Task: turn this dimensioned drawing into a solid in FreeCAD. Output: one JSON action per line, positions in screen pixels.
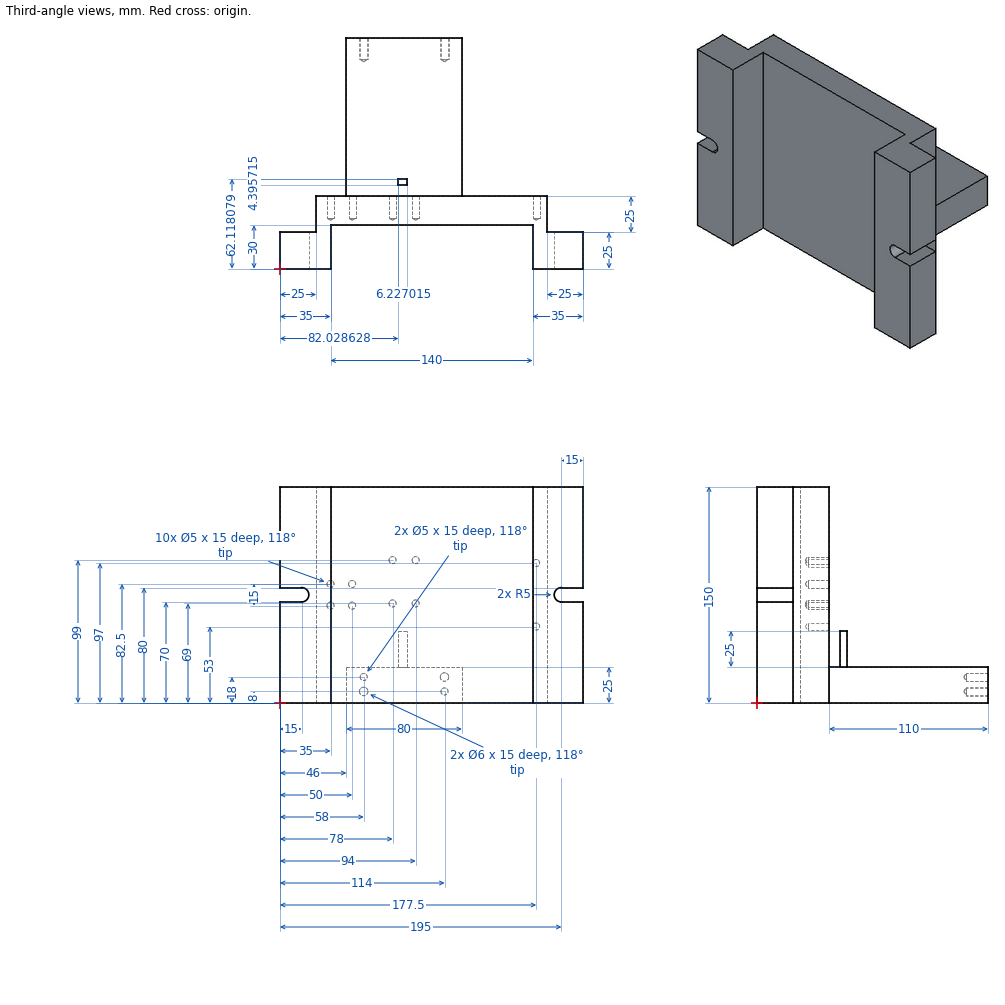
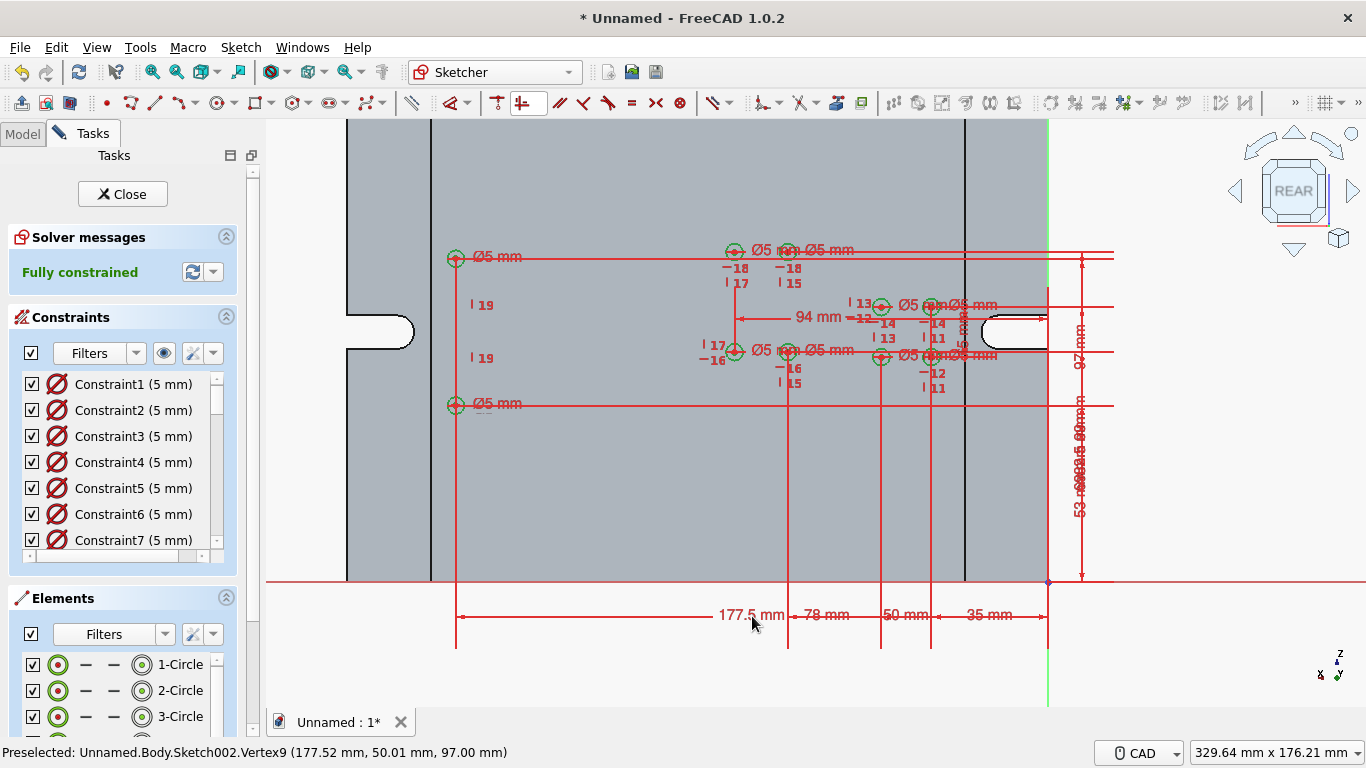
{"action": "left_click", "coordinate": [123, 194]}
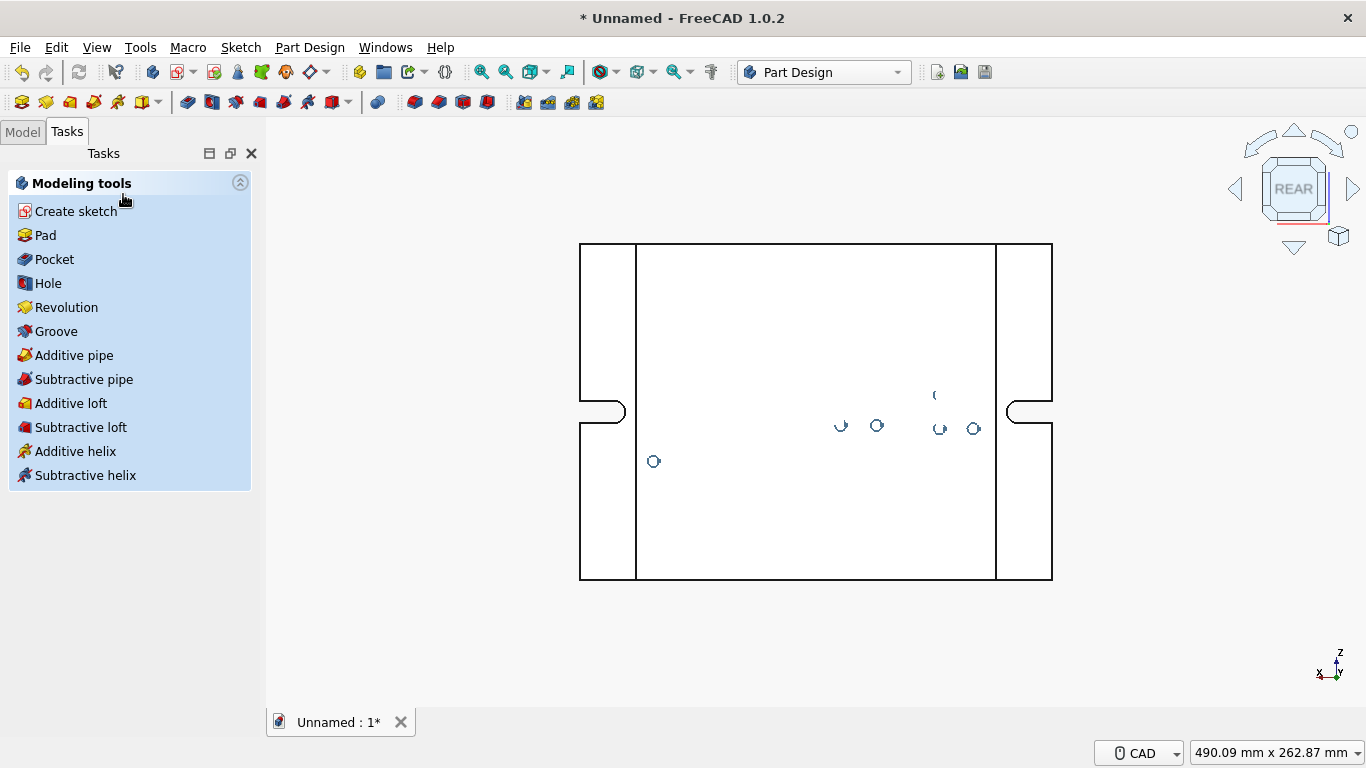
{"action": "left_click", "coordinate": [212, 102]}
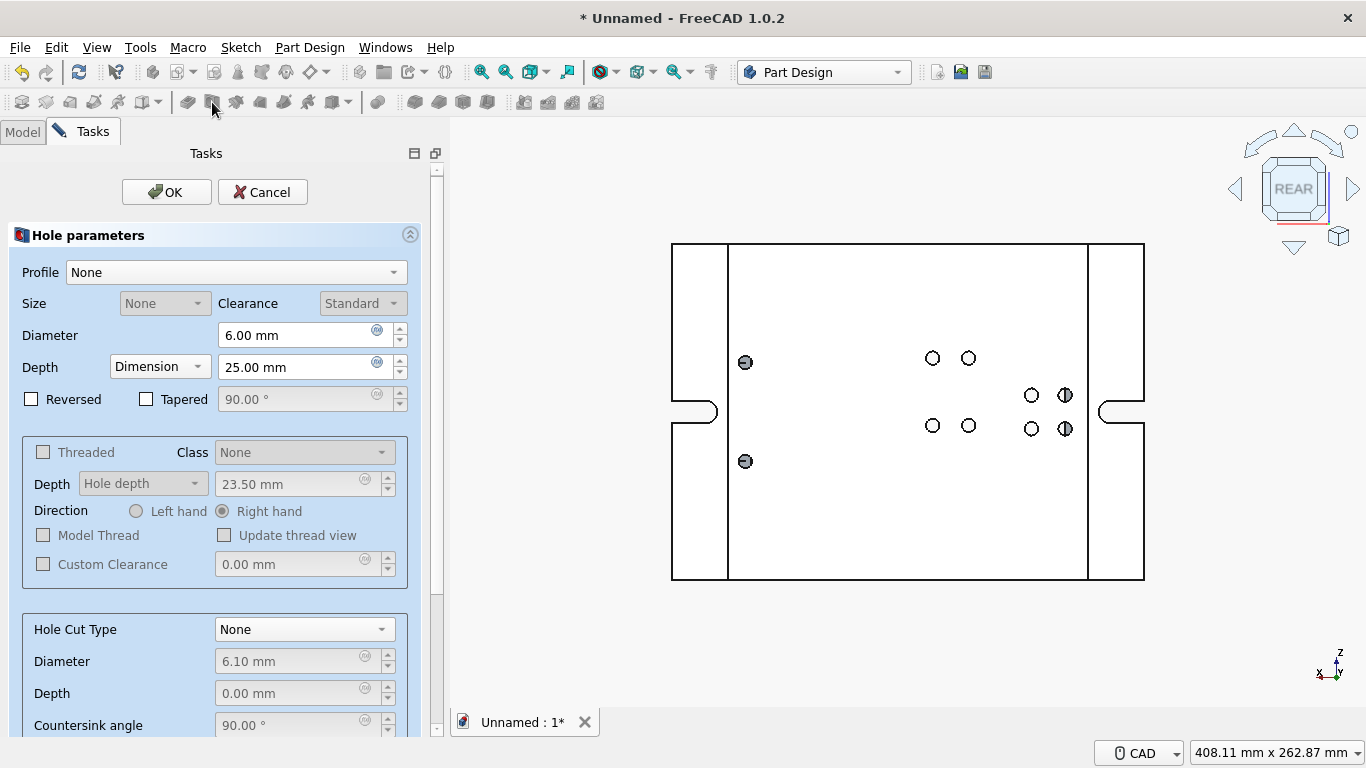
{"action": "triple_click", "coordinate": [305, 335]}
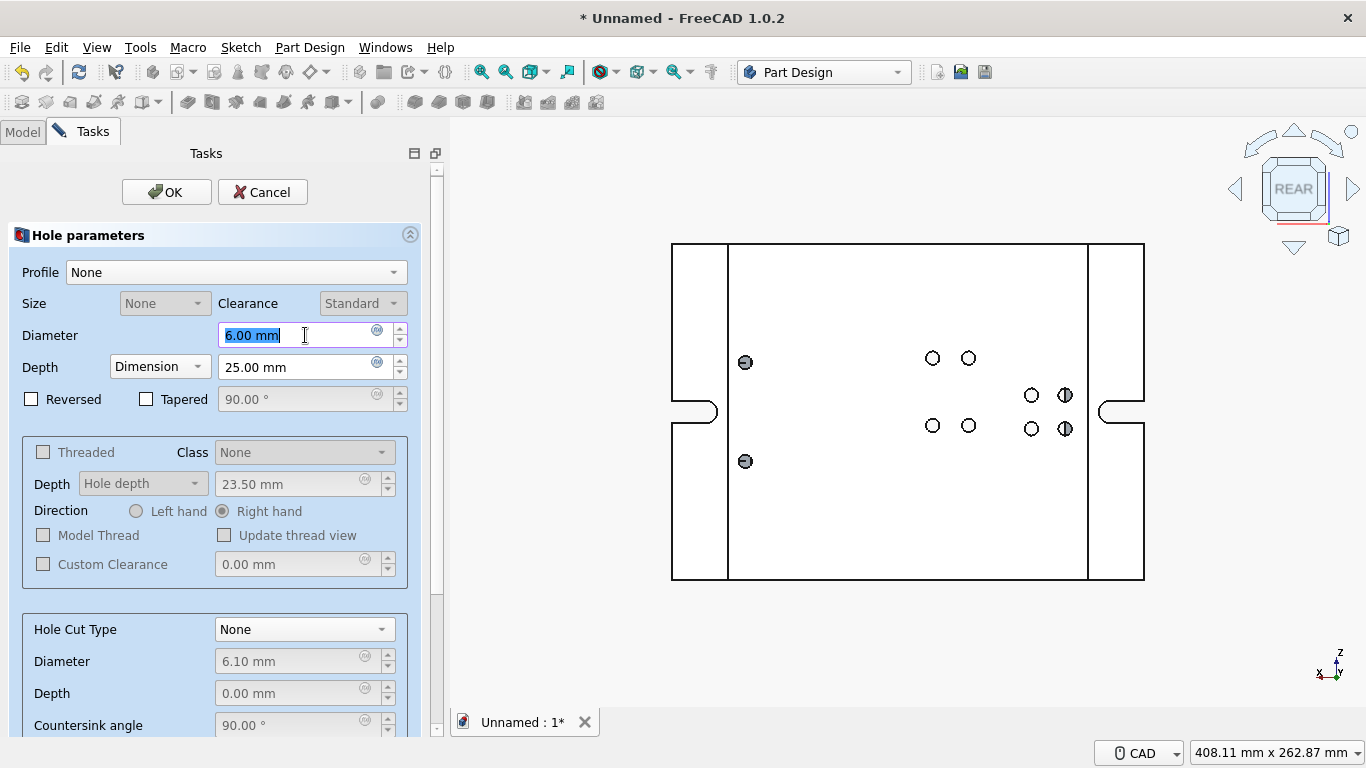
{"action": "type", "text": "5"}
{"action": "key", "text": "Tab"}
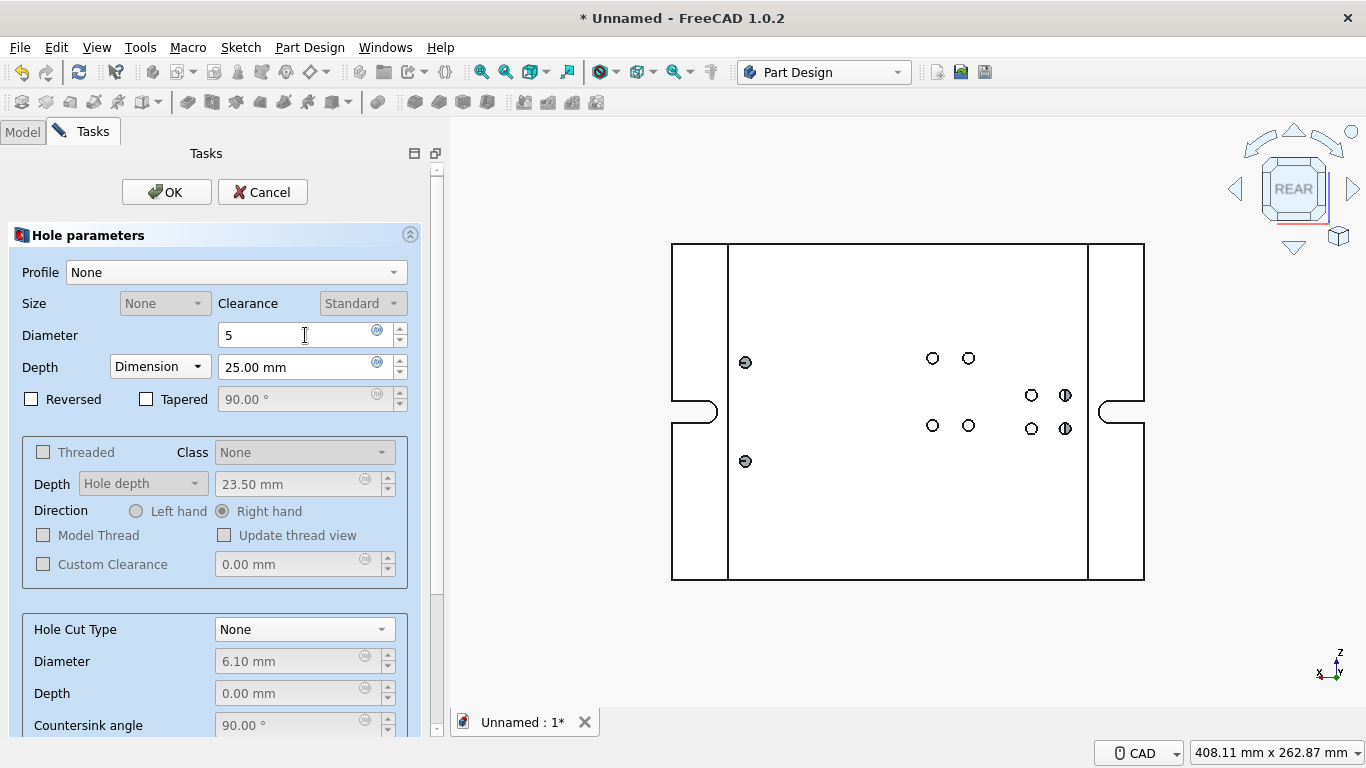
{"action": "triple_click", "coordinate": [305, 367]}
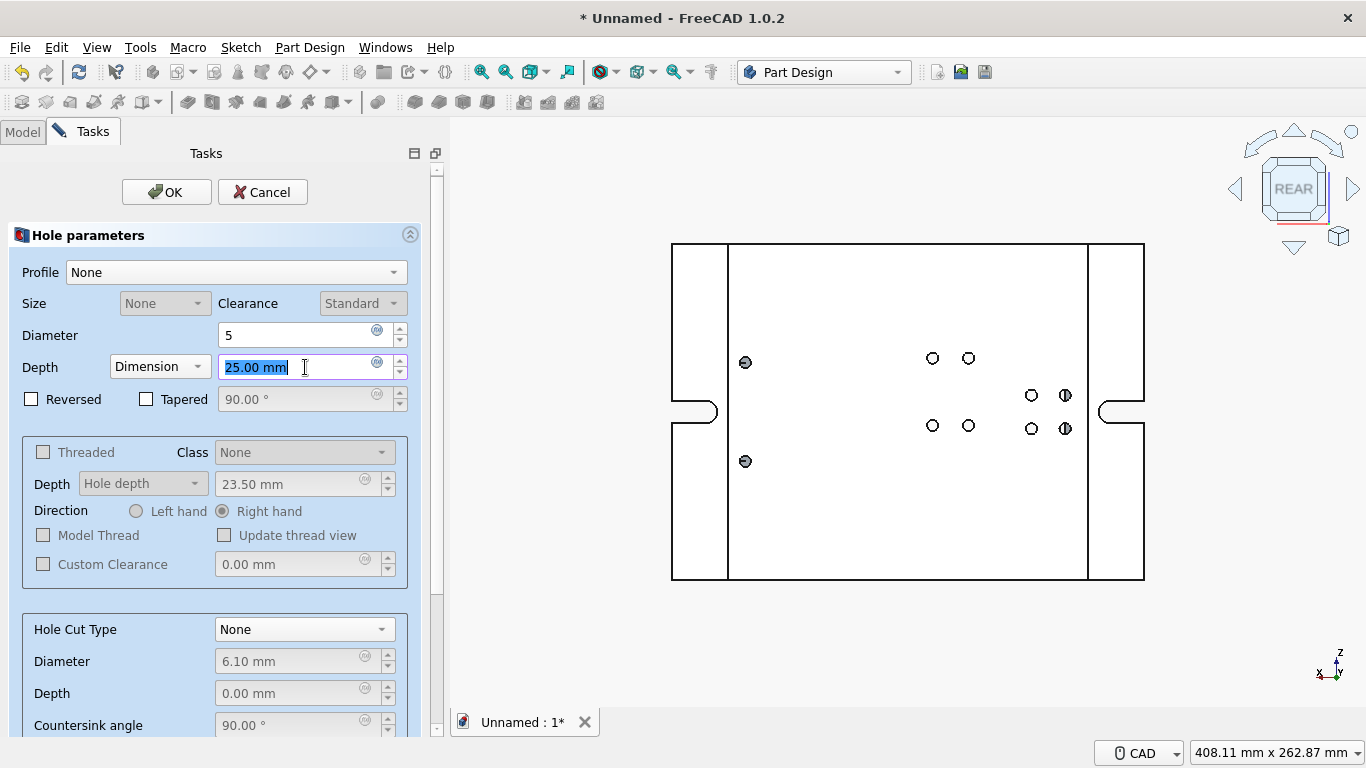
{"action": "type", "text": "15"}
{"action": "key", "text": "Tab"}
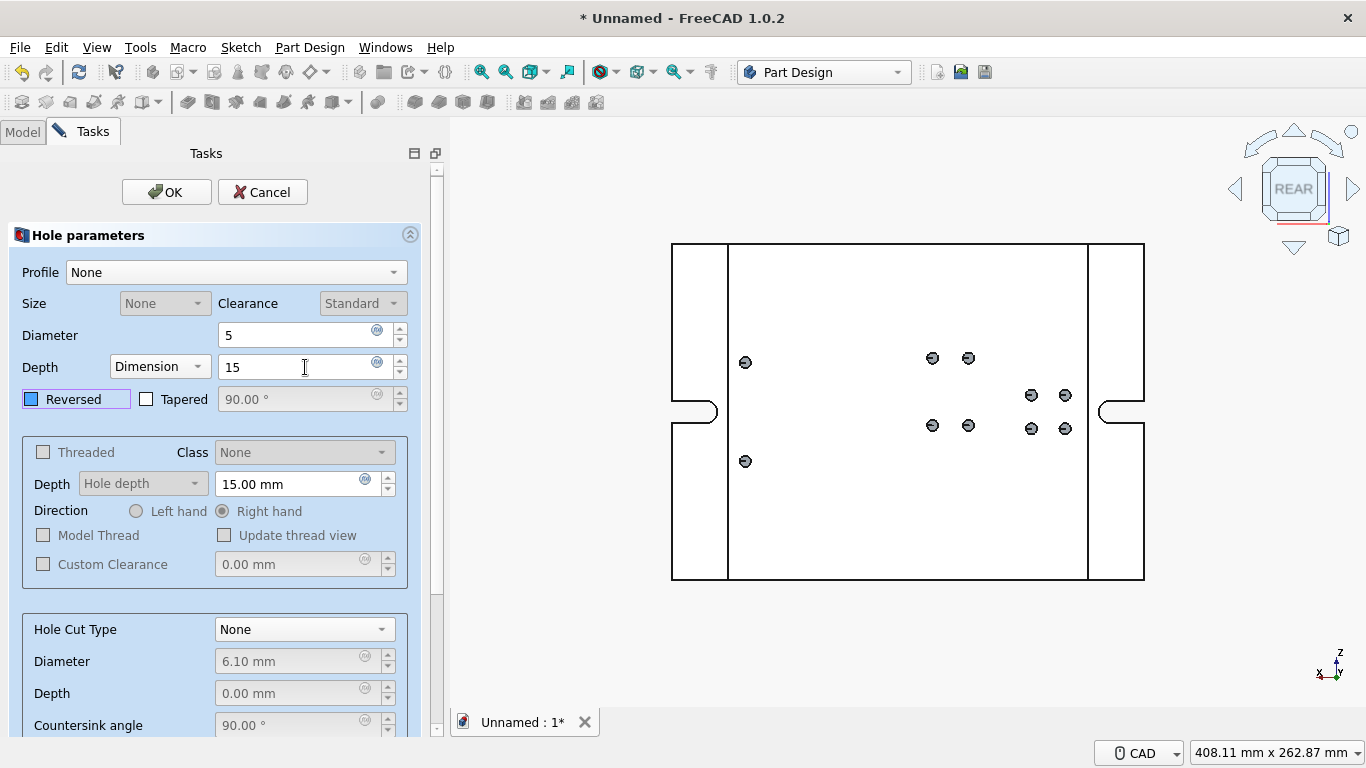
{"action": "left_click", "coordinate": [167, 192]}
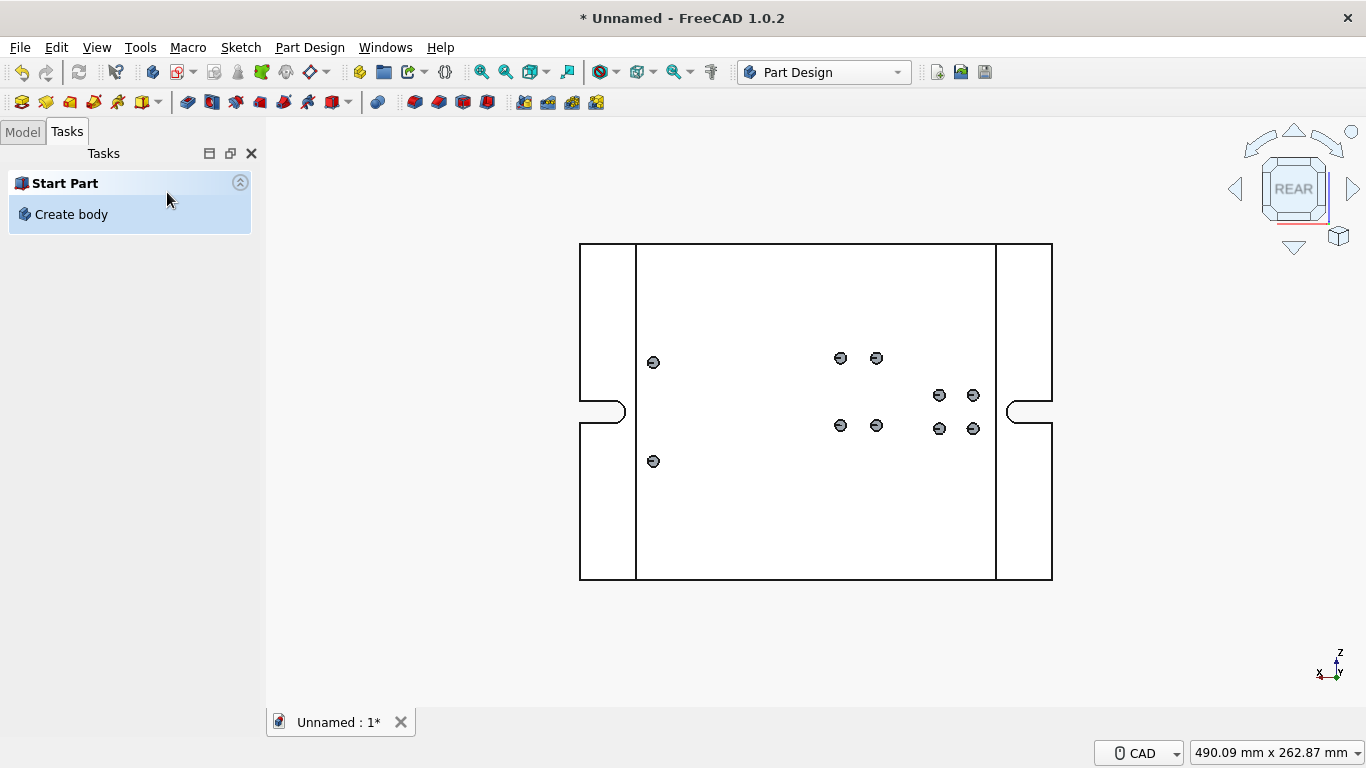
{"action": "left_click", "coordinate": [765, 459]}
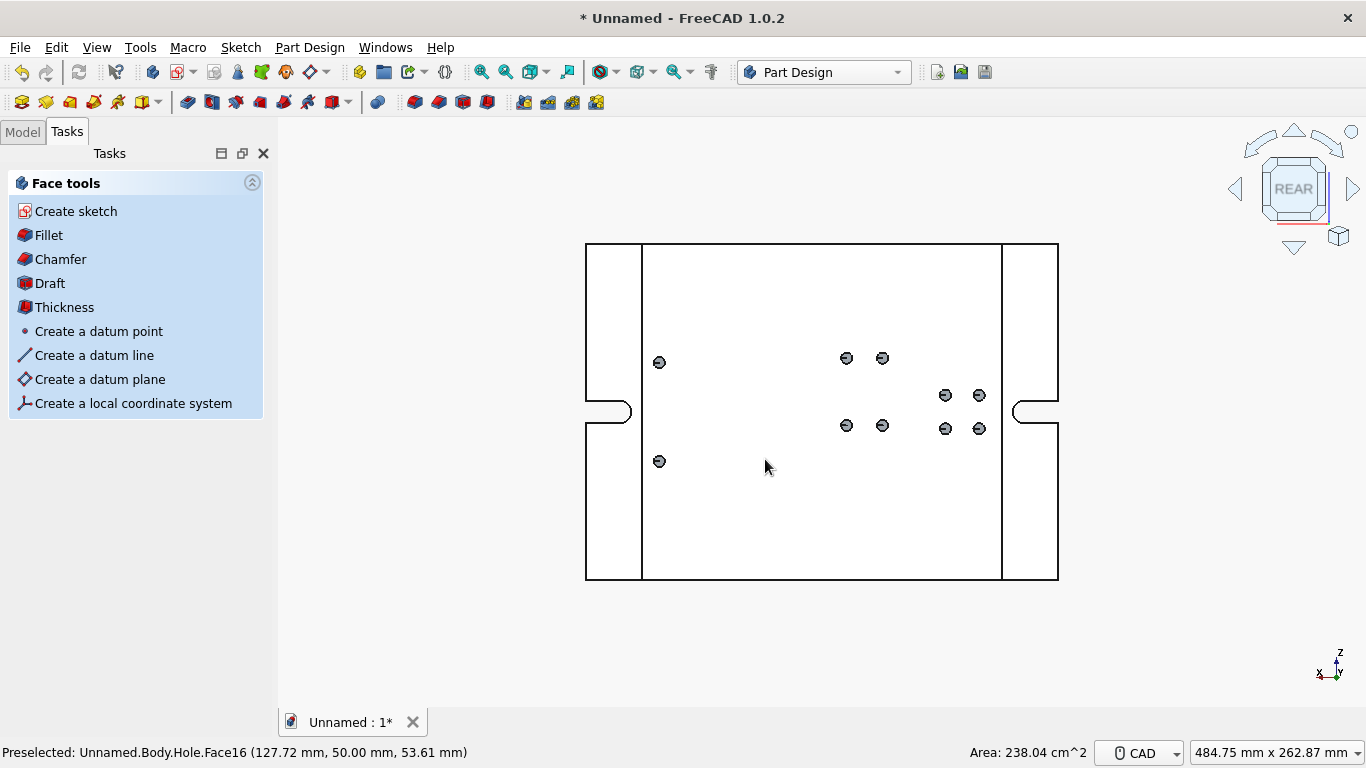
{"action": "left_click", "coordinate": [178, 72]}